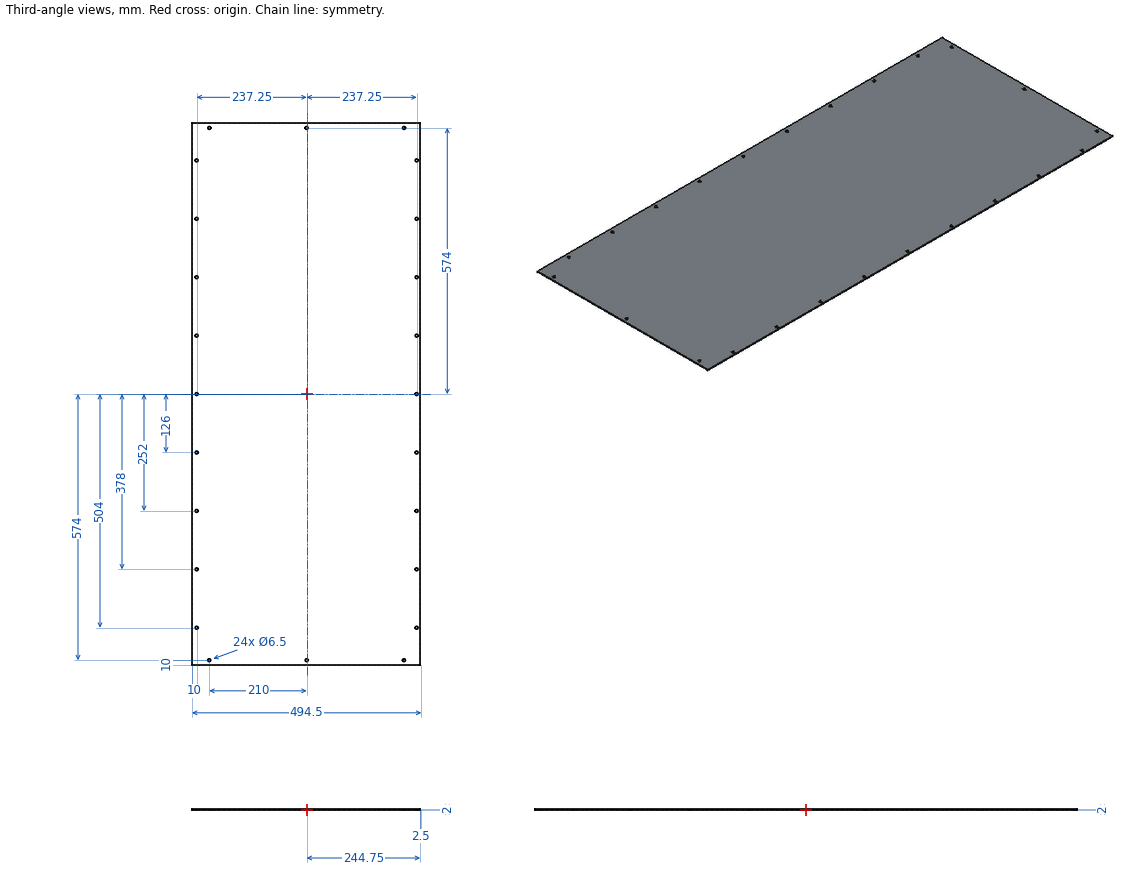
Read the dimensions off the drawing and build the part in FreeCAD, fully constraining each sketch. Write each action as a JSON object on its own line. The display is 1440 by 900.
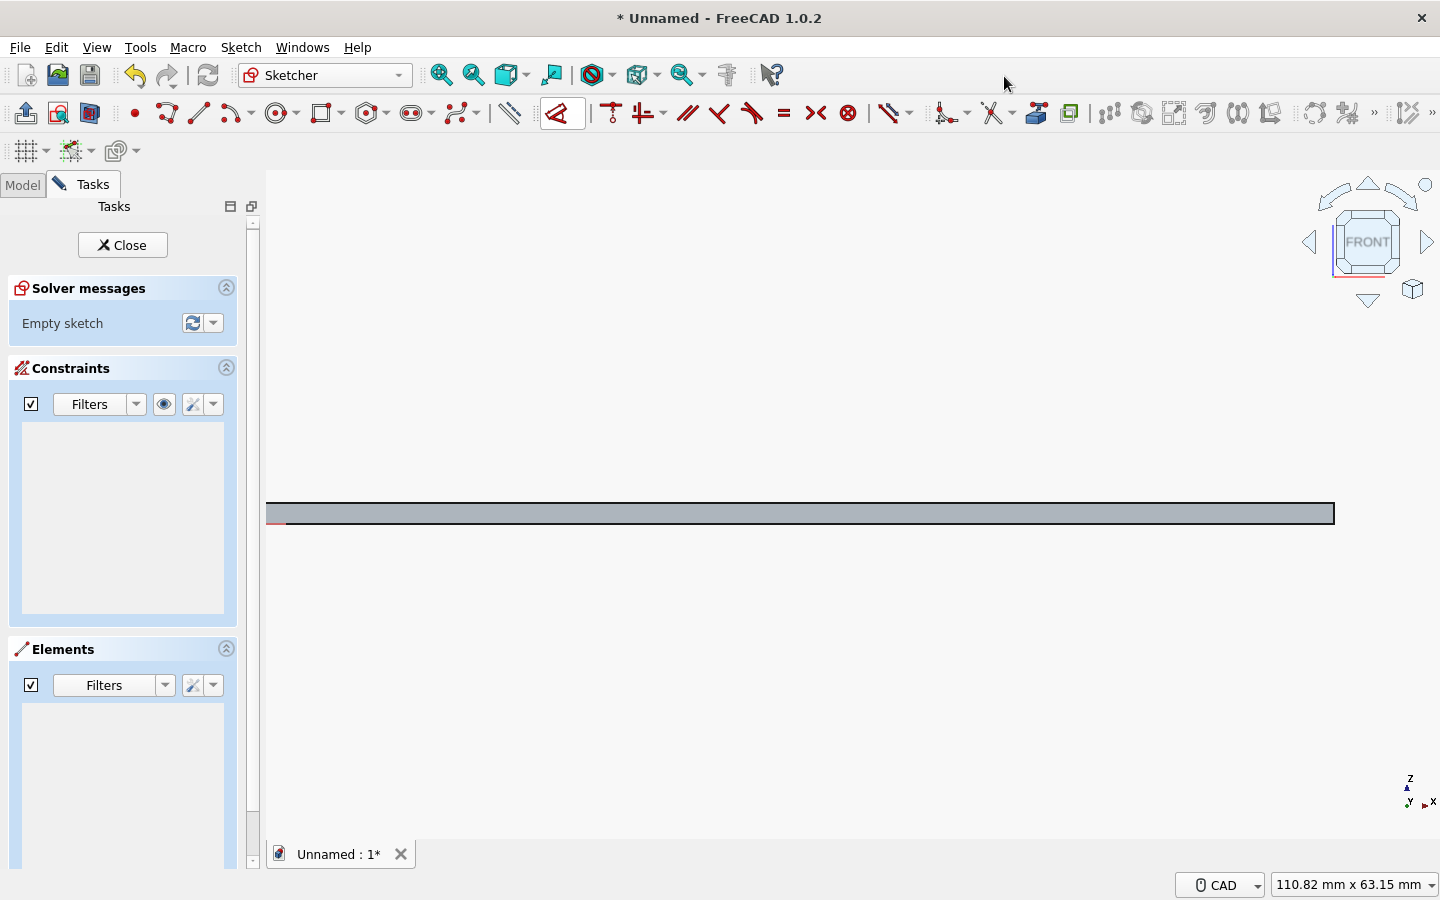
{"action": "scroll", "coordinate": [784, 504], "scroll_direction": "down", "scroll_amount": 5}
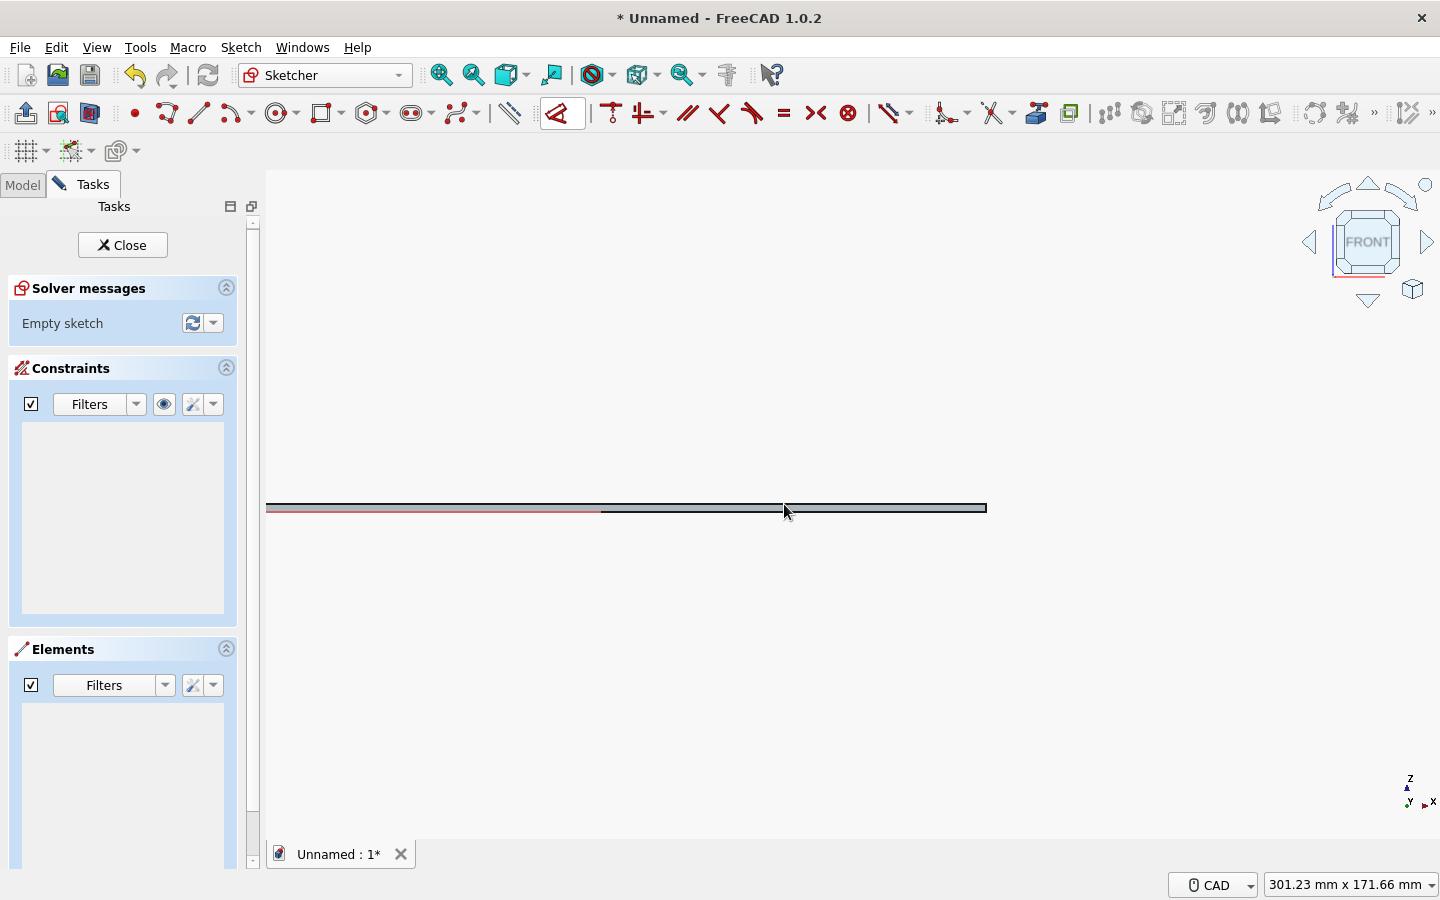
{"action": "scroll", "coordinate": [992, 508], "scroll_direction": "up", "scroll_amount": 15}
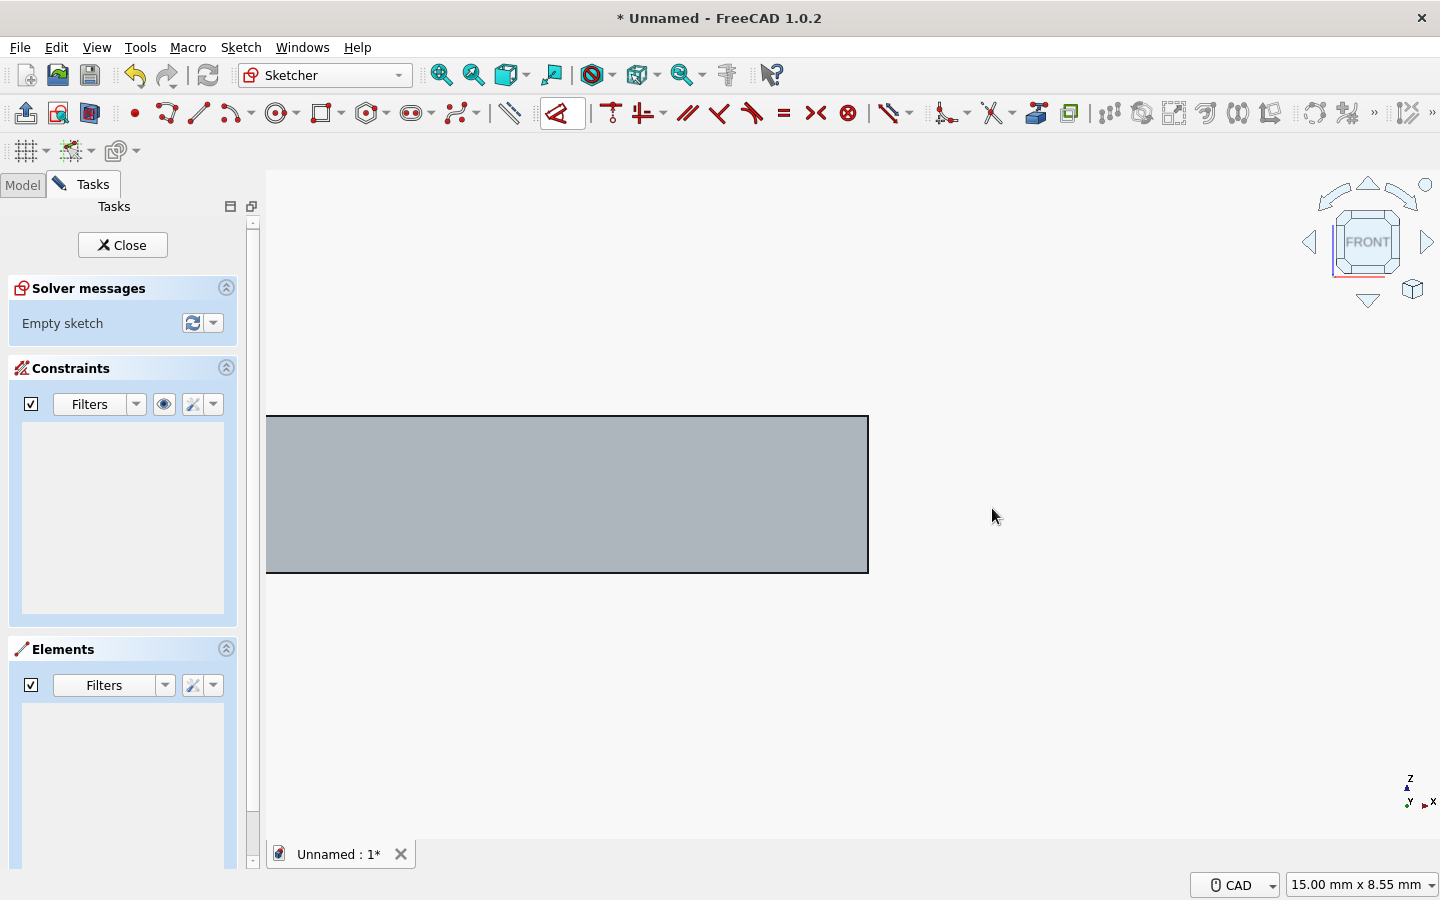
{"action": "scroll", "coordinate": [762, 489], "scroll_direction": "up", "scroll_amount": 5}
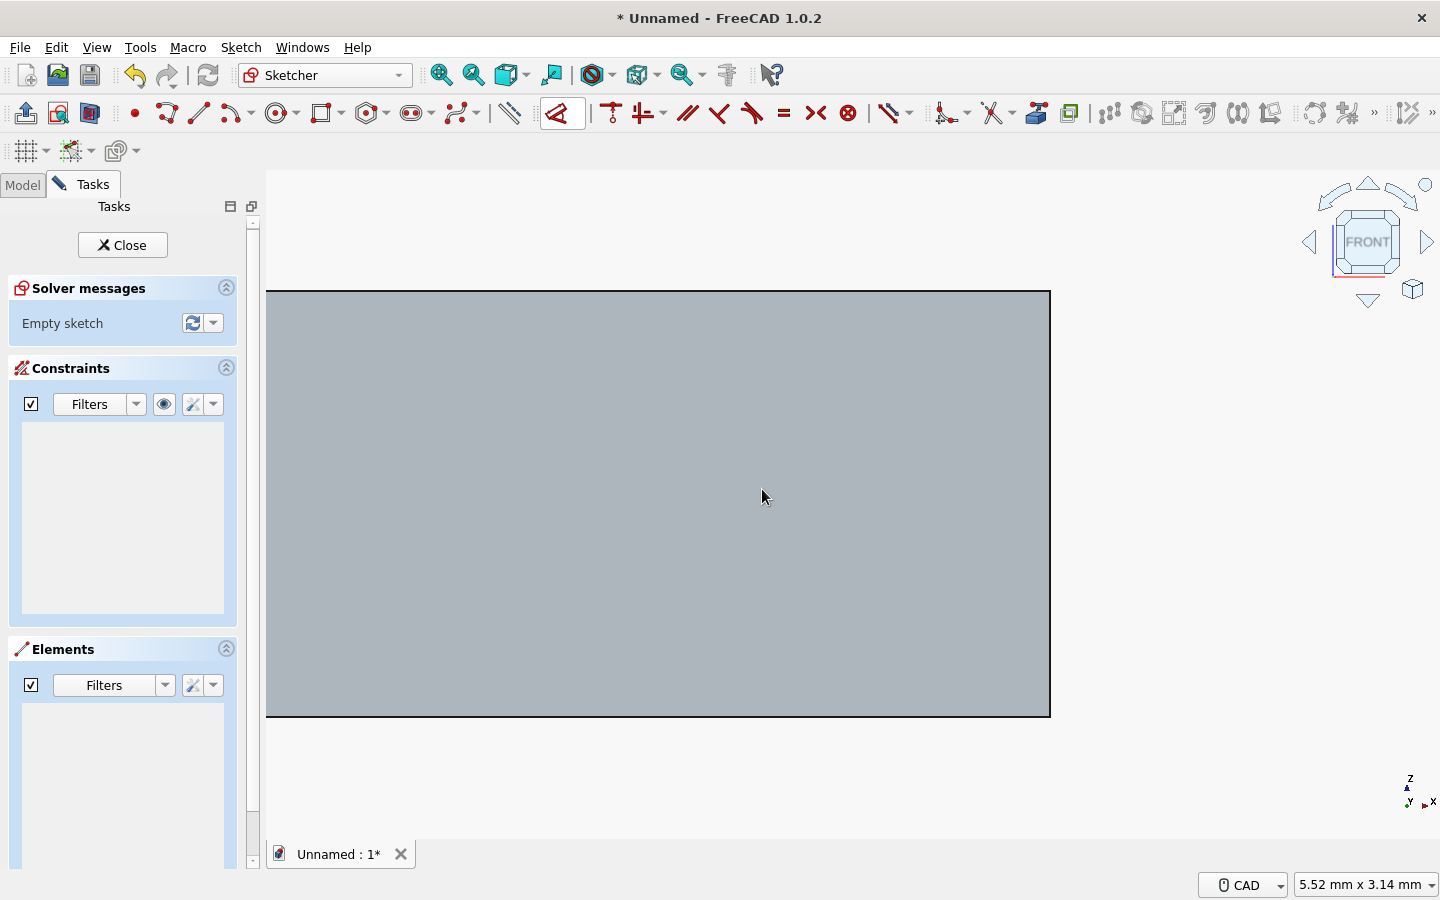
{"action": "left_click", "coordinate": [322, 114]}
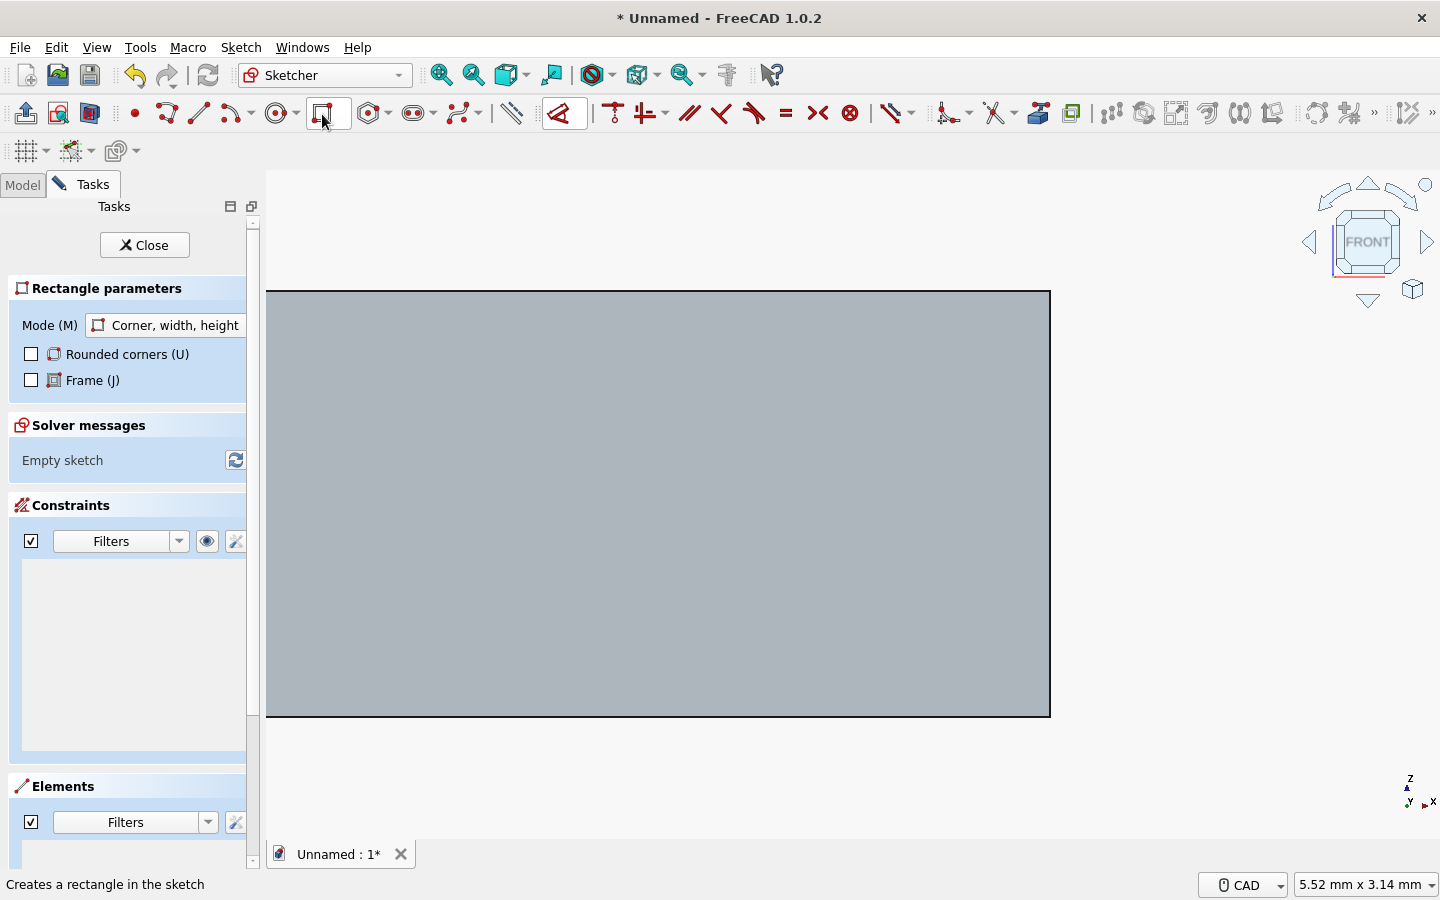
{"action": "left_click", "coordinate": [519, 291]}
{"action": "left_click", "coordinate": [1050, 717]}
{"action": "key", "text": "Escape"}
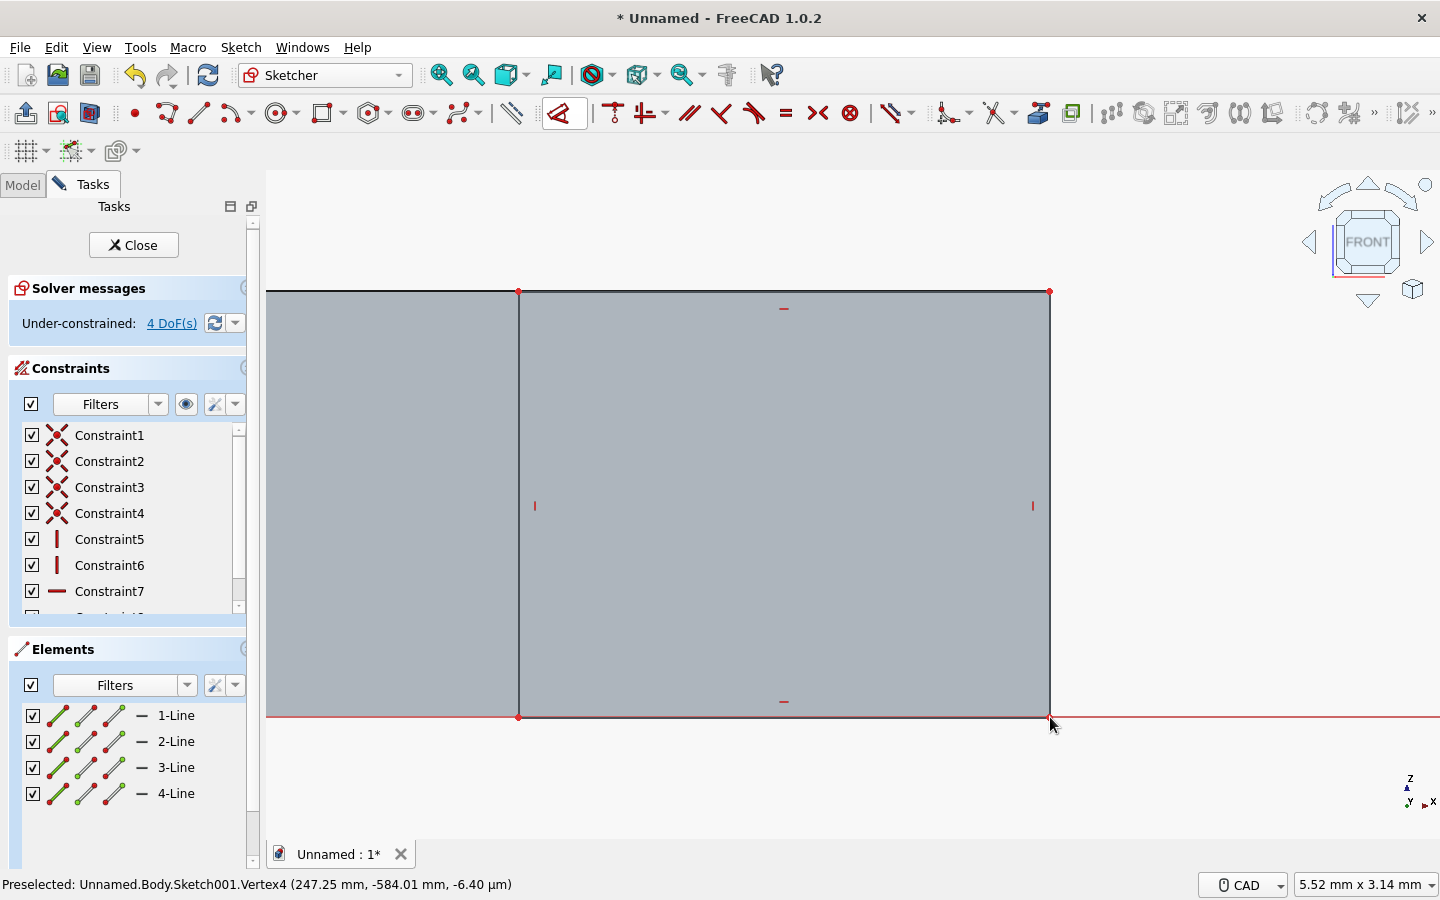
{"action": "left_click", "coordinate": [519, 718]}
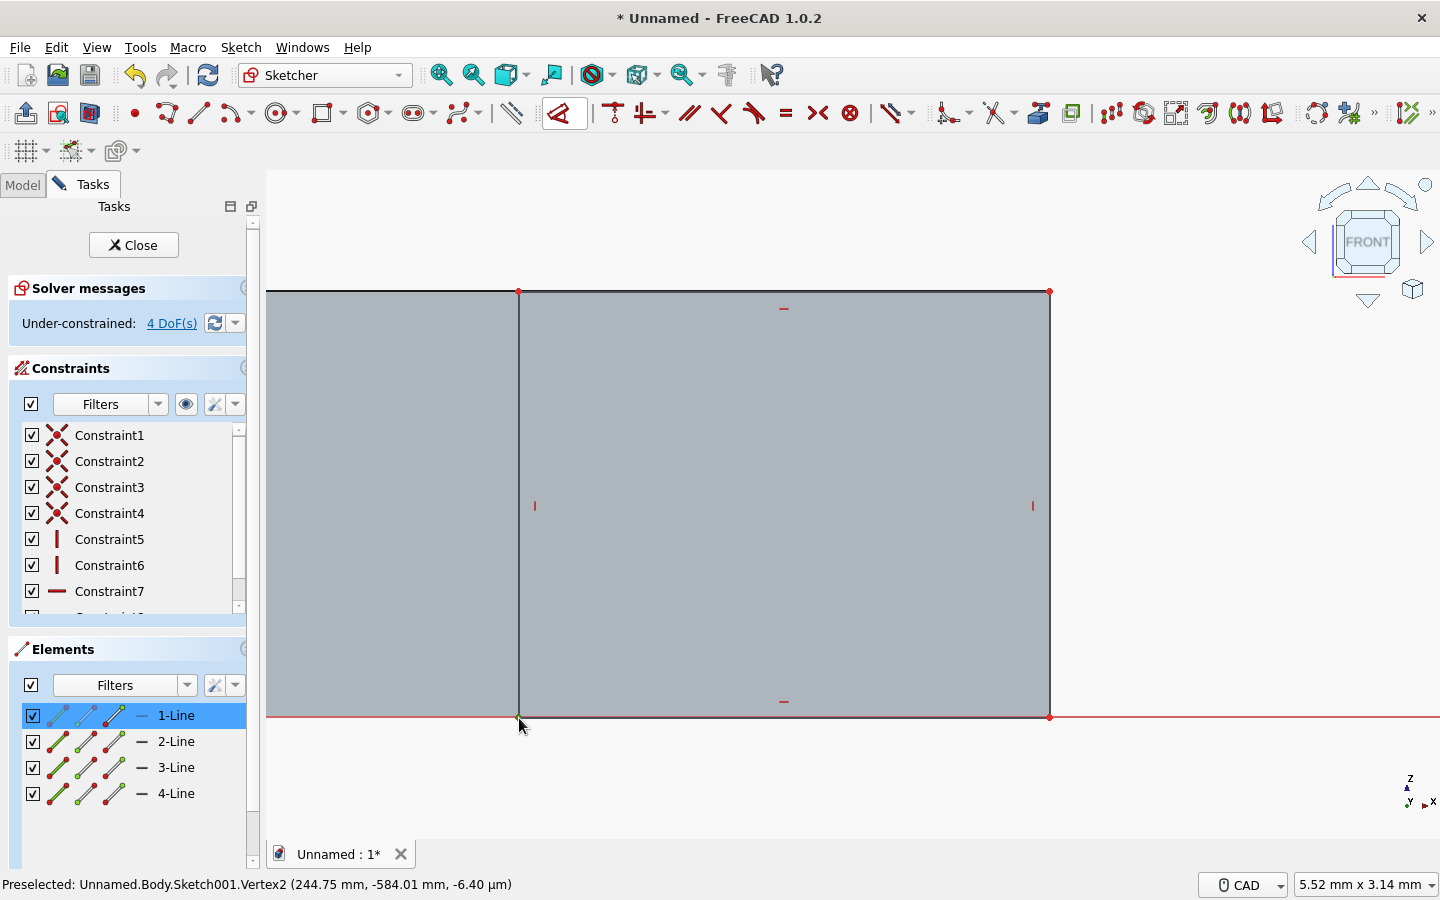
{"action": "left_click", "coordinate": [364, 717]}